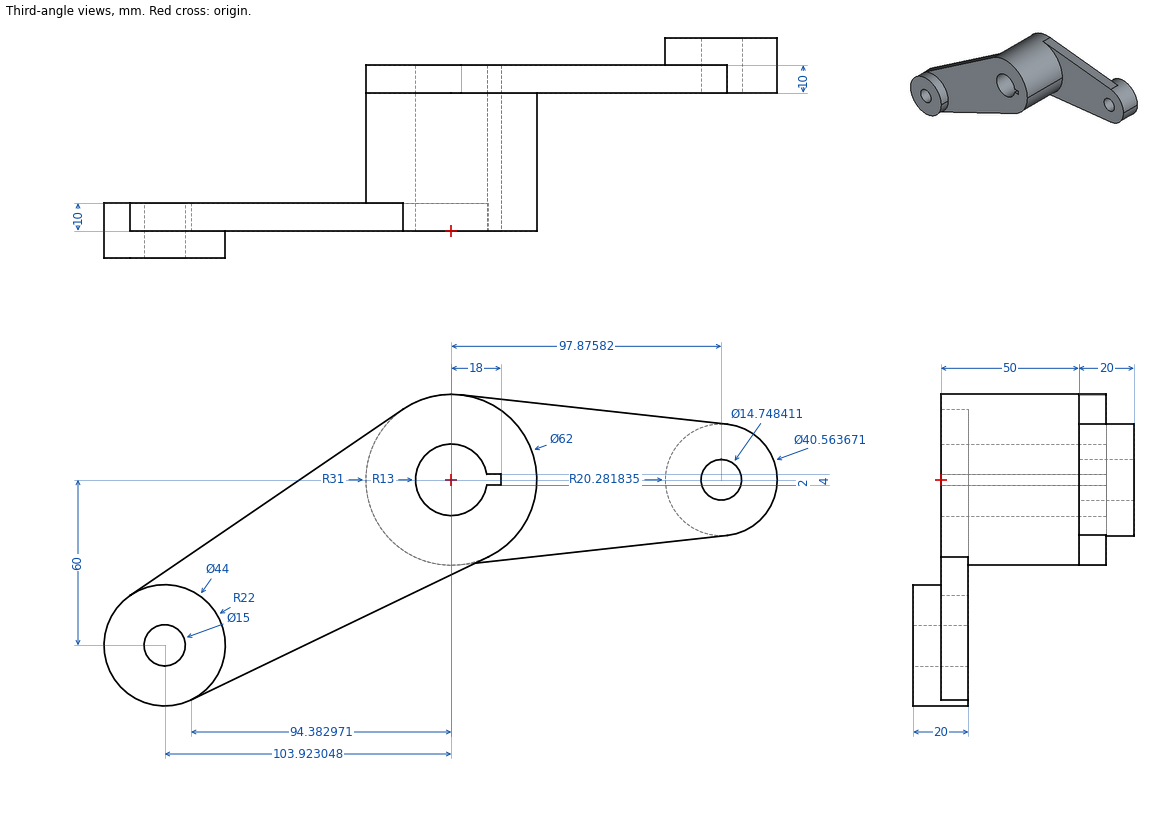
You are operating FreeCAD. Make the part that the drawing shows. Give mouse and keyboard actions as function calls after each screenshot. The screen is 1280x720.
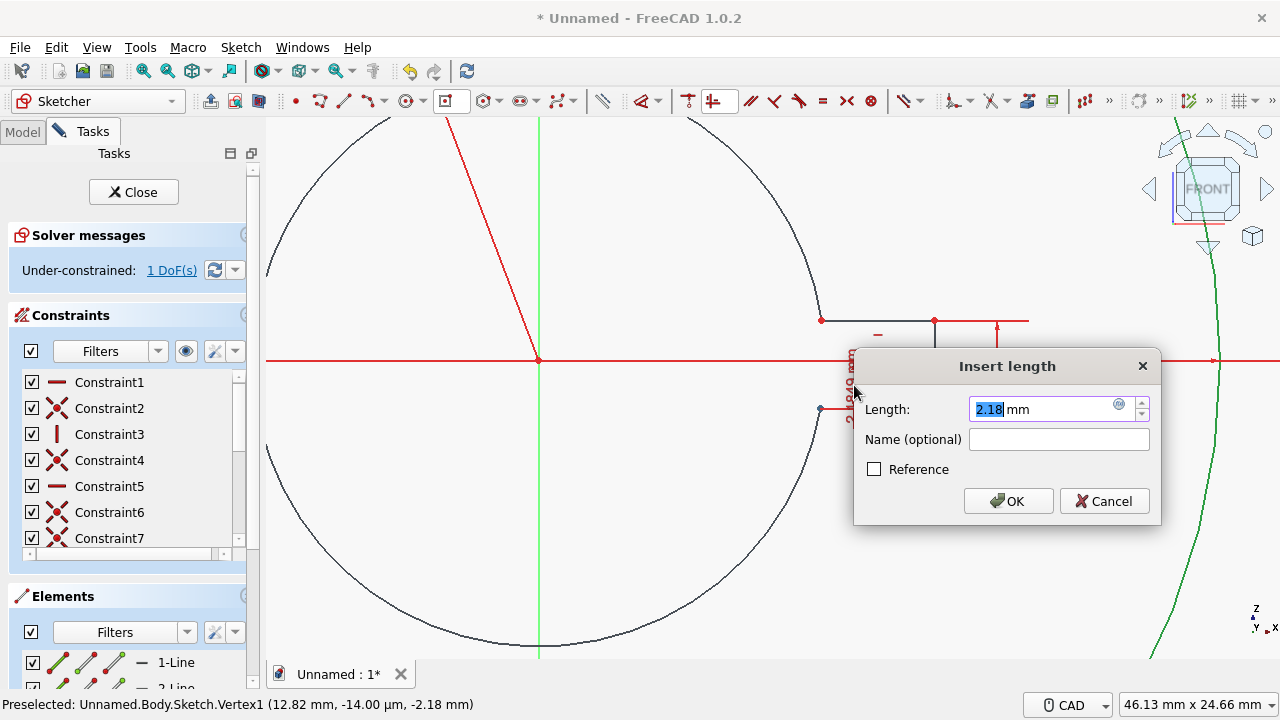
text(2)
key(Return)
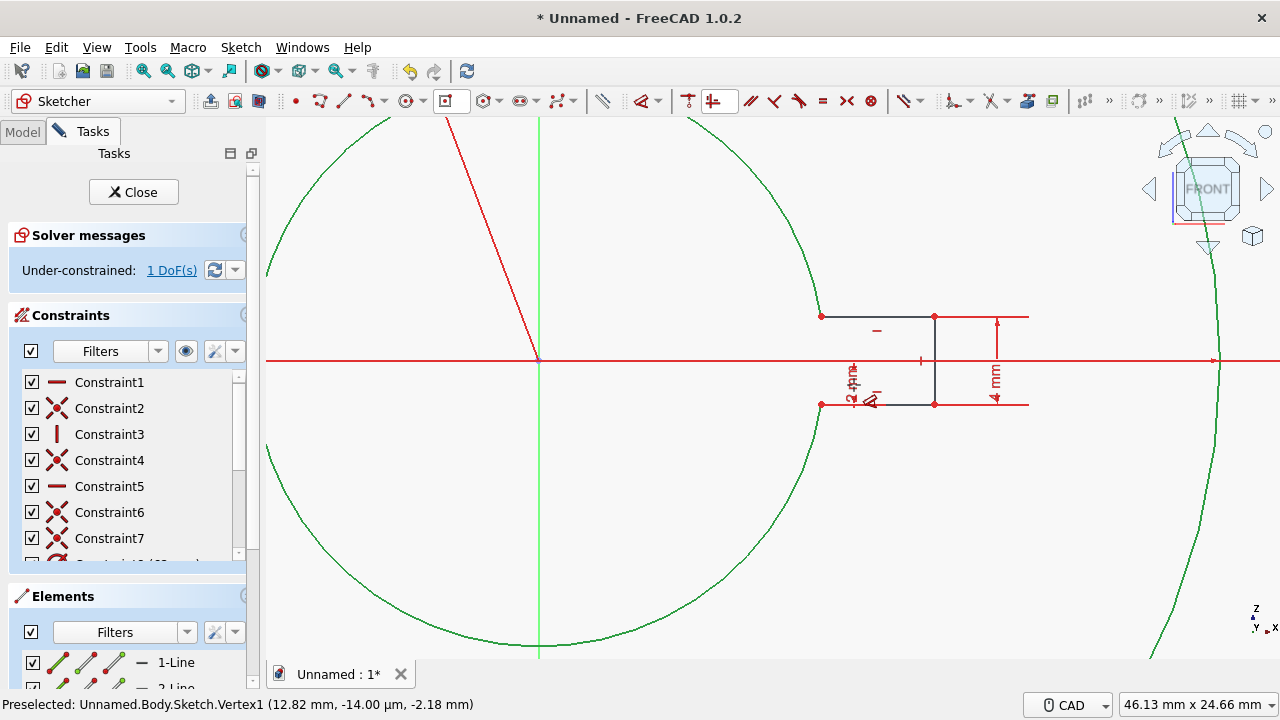
scroll(759, 397, down, 7)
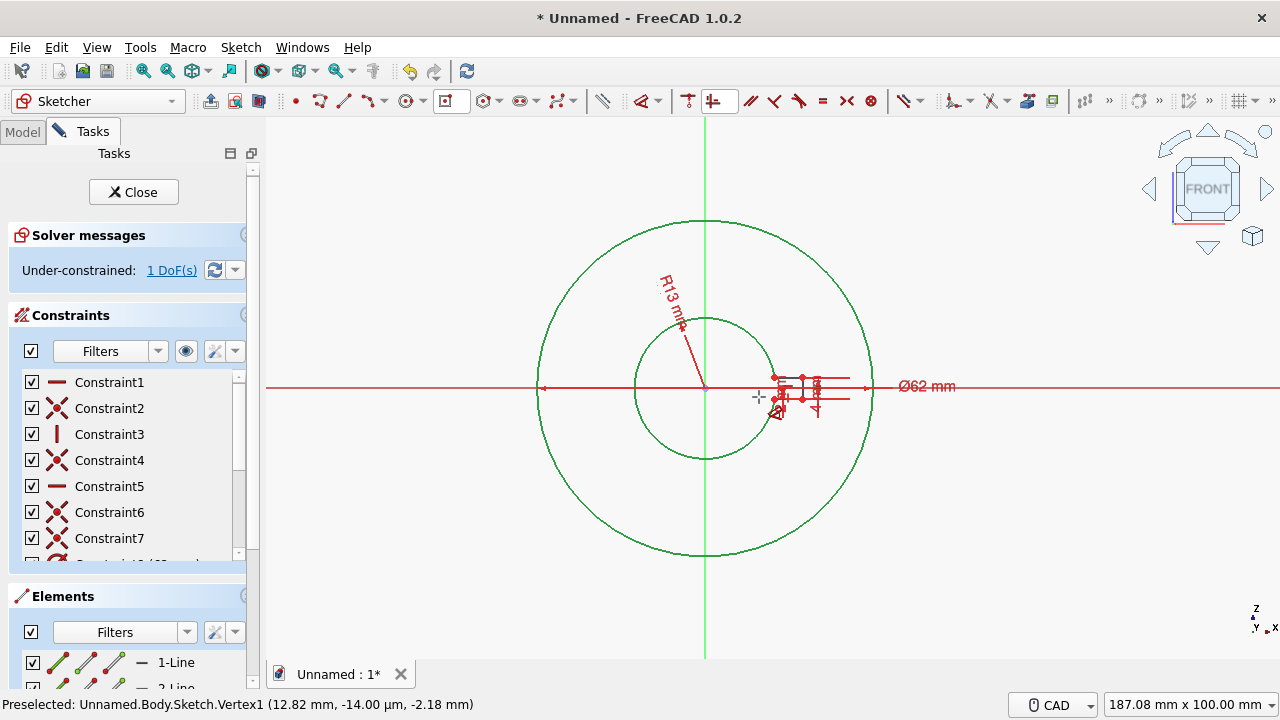
click(803, 399)
click(731, 433)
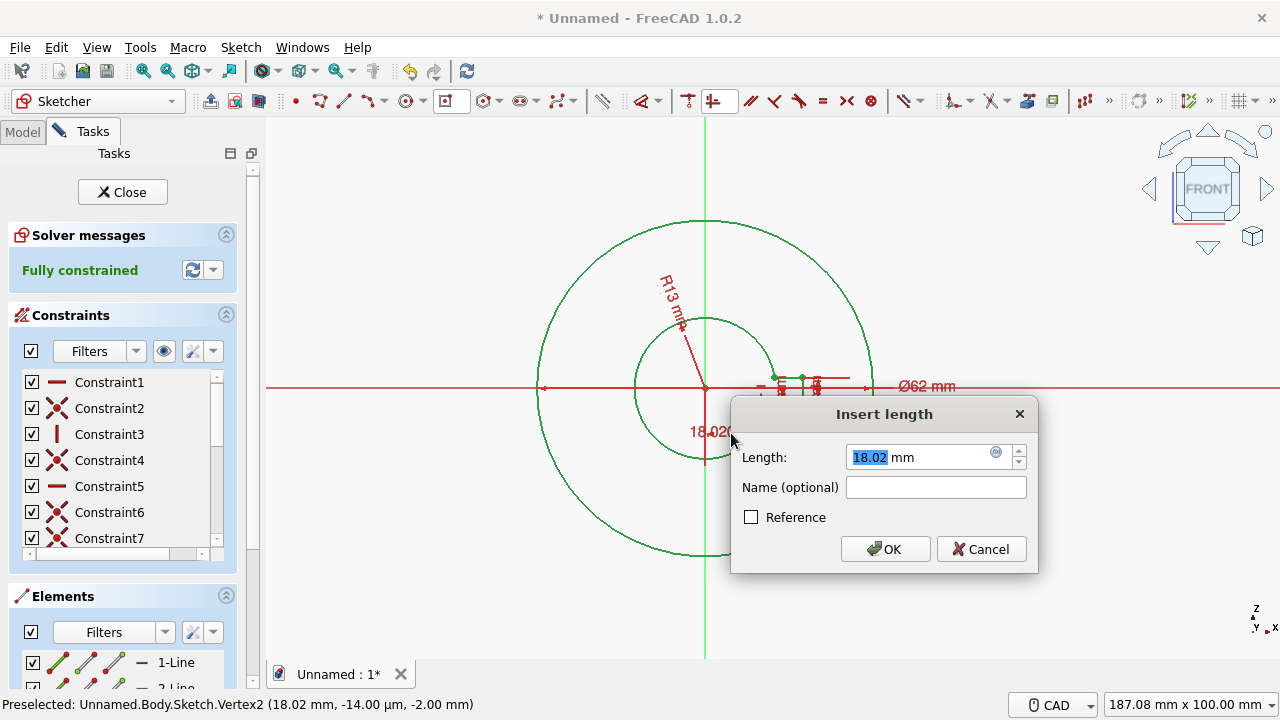
text(18)
key(Return)
key(Escape)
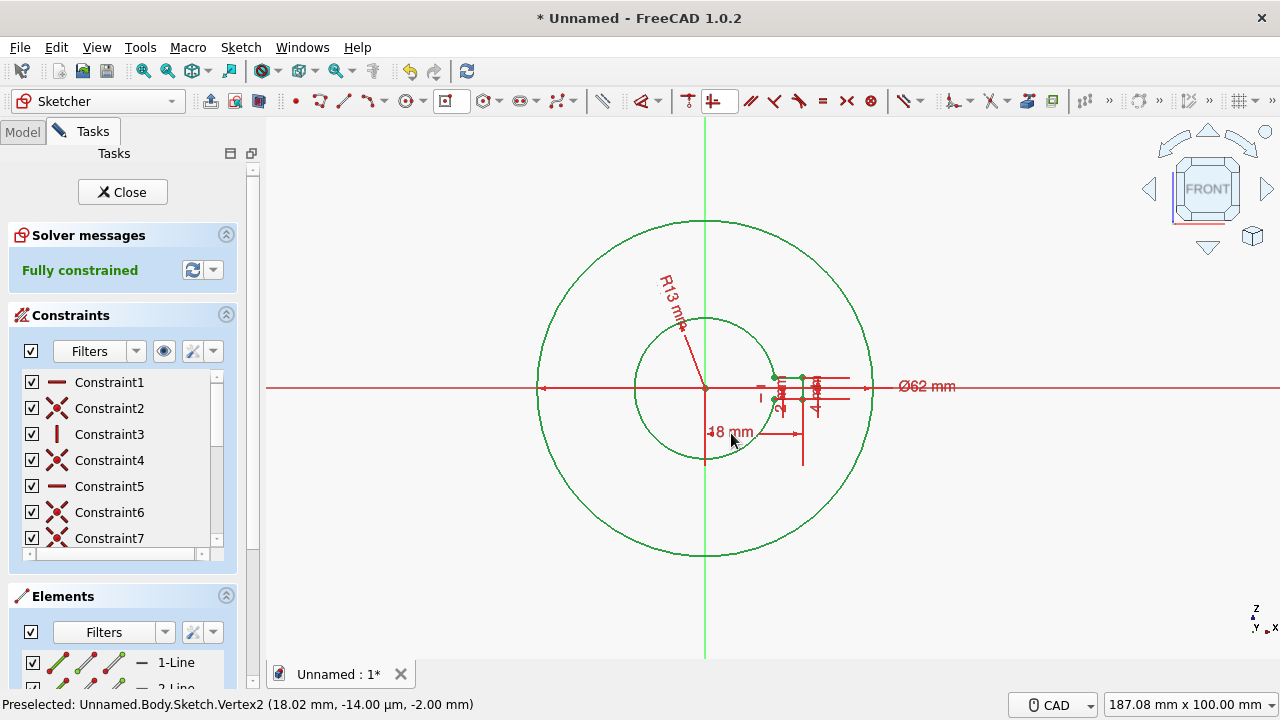
click(123, 192)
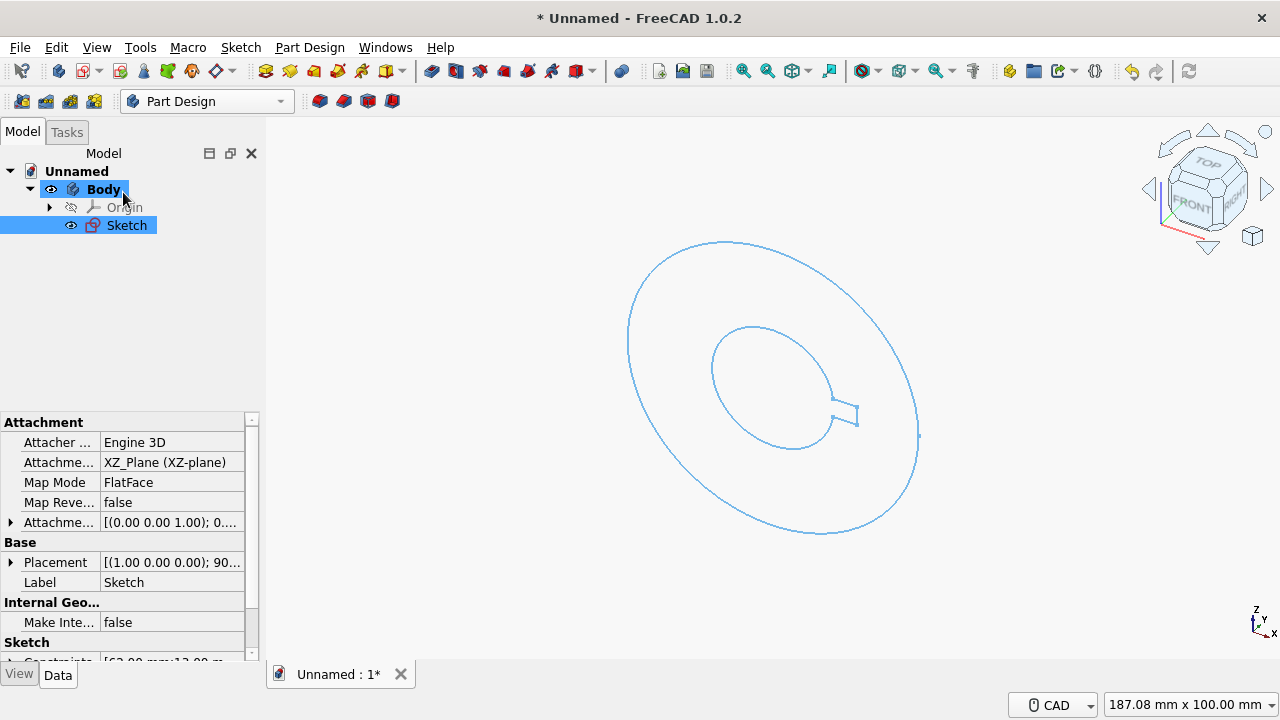
click(266, 72)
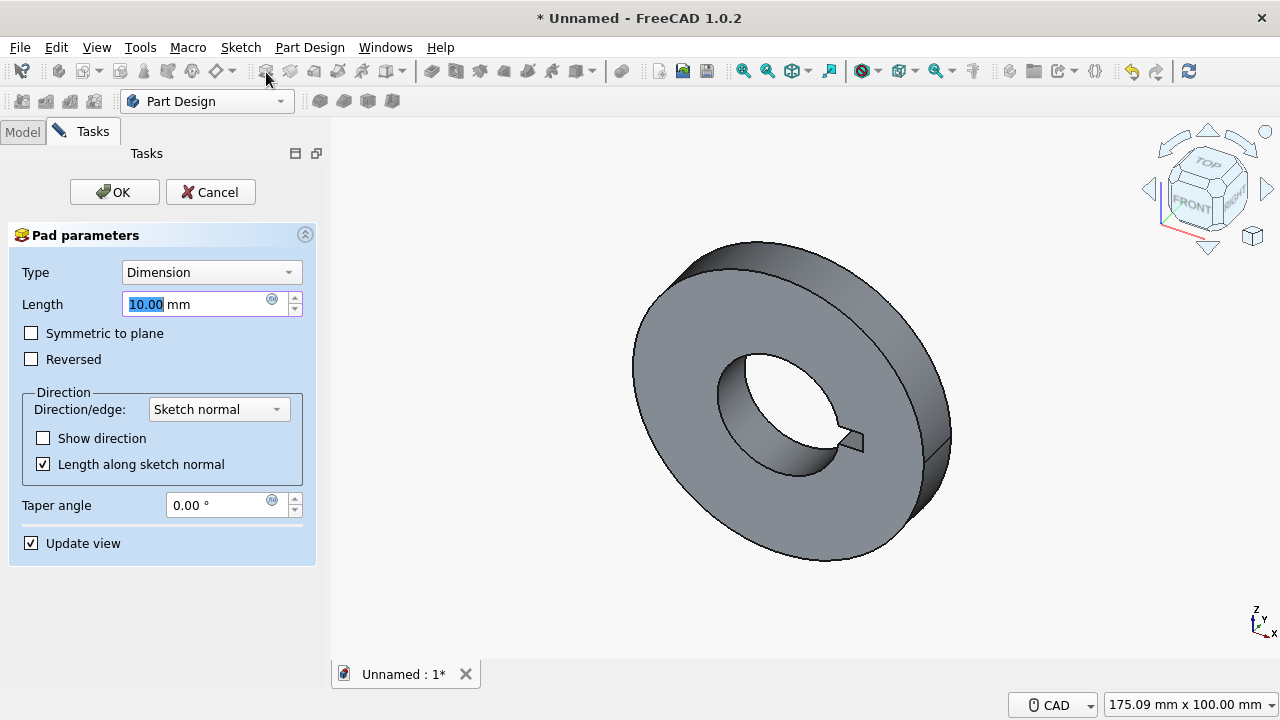
text(50)
key(Tab)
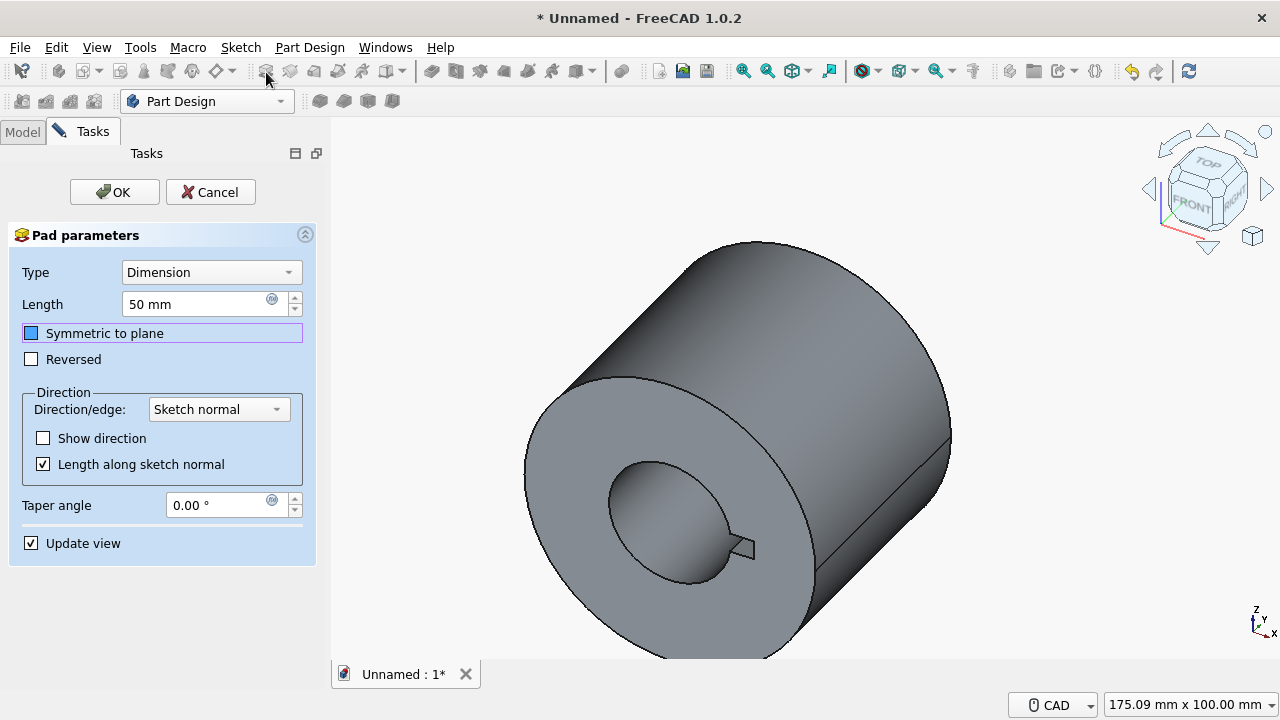
click(30, 359)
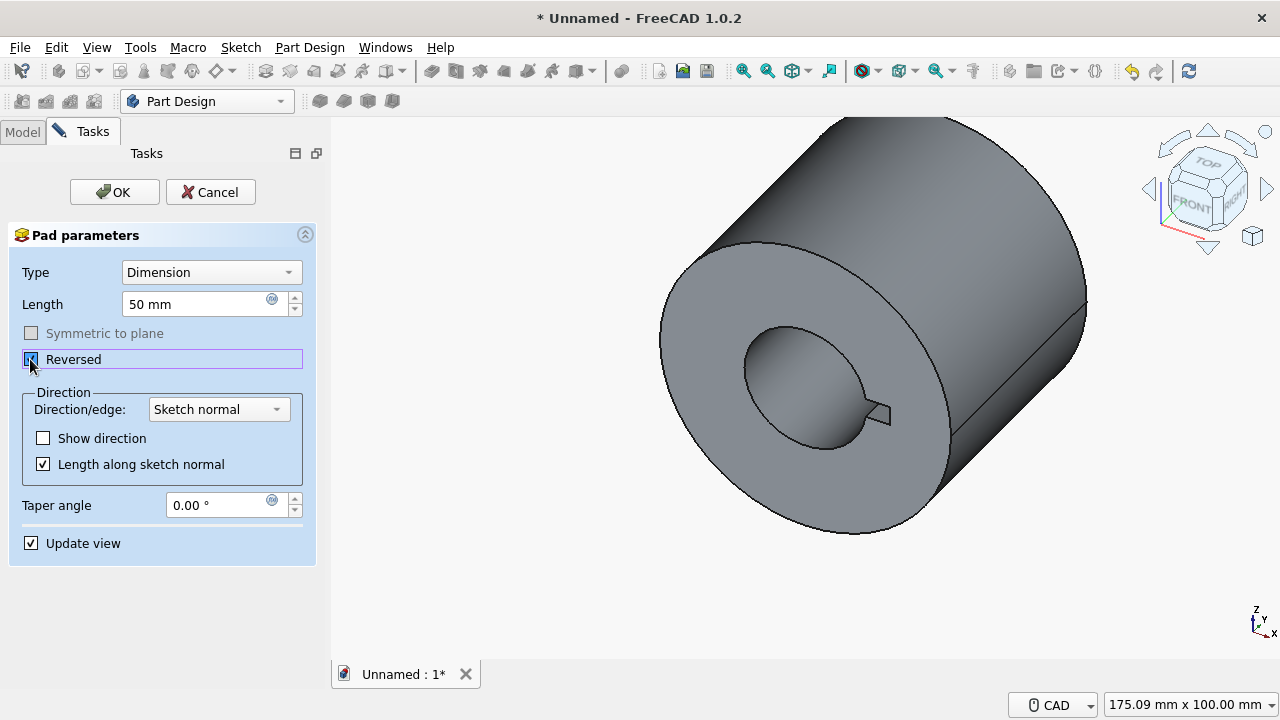
click(115, 192)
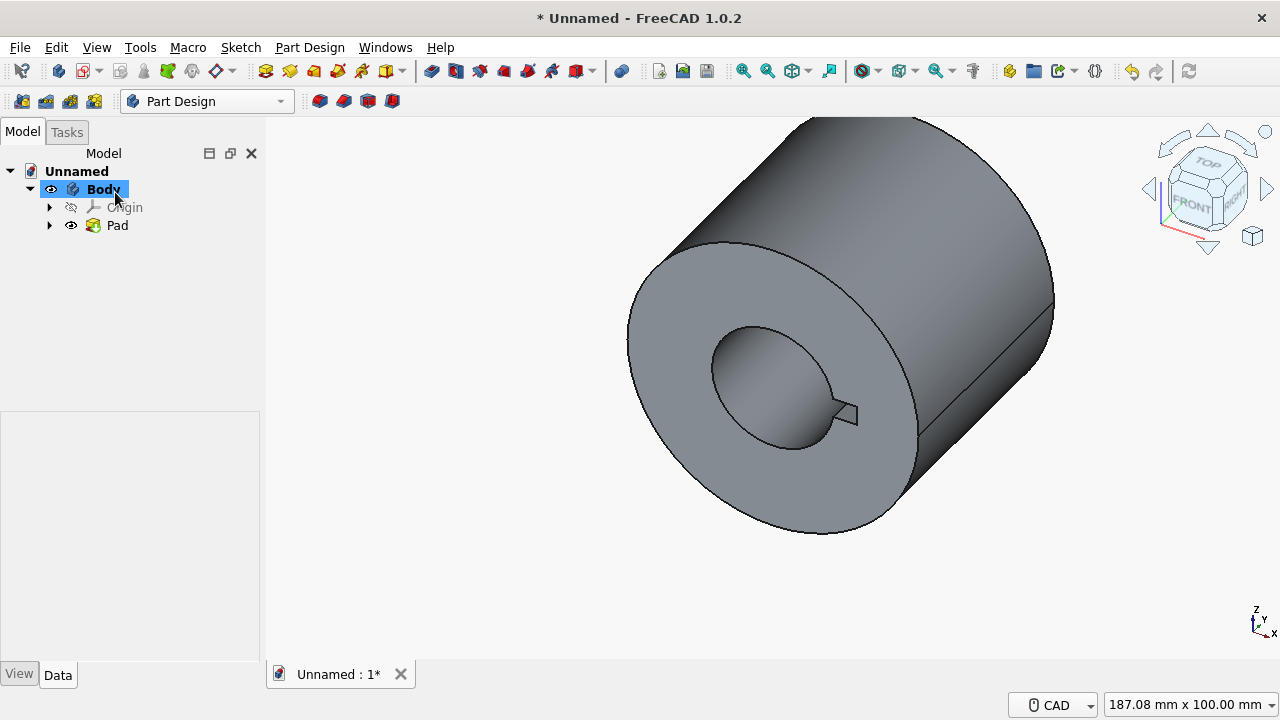
click(744, 72)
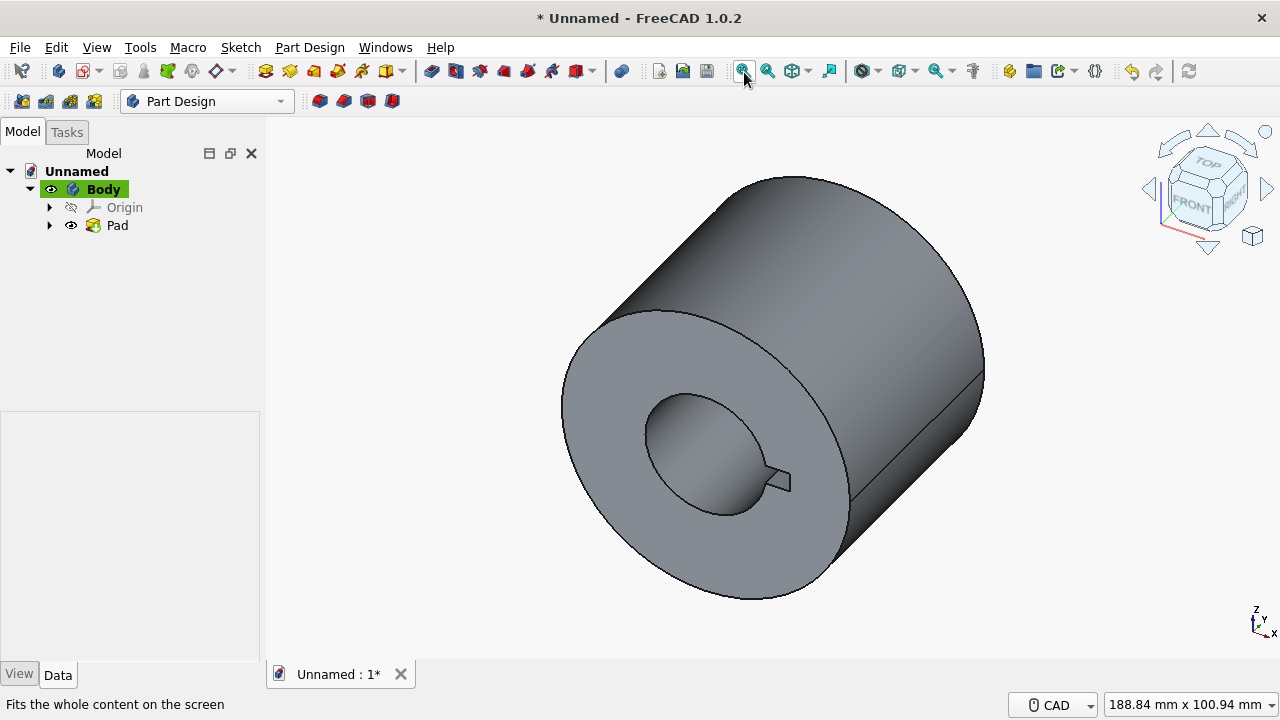
key(4)